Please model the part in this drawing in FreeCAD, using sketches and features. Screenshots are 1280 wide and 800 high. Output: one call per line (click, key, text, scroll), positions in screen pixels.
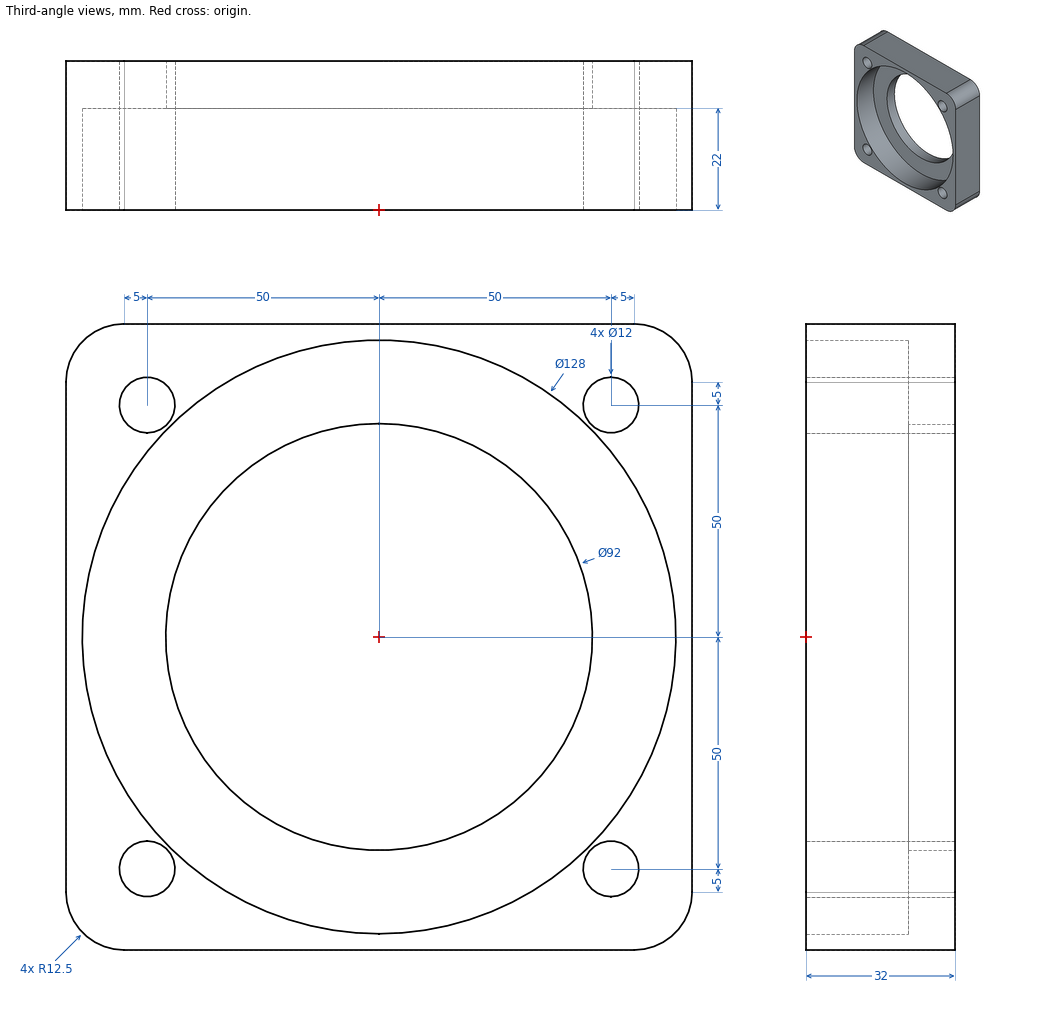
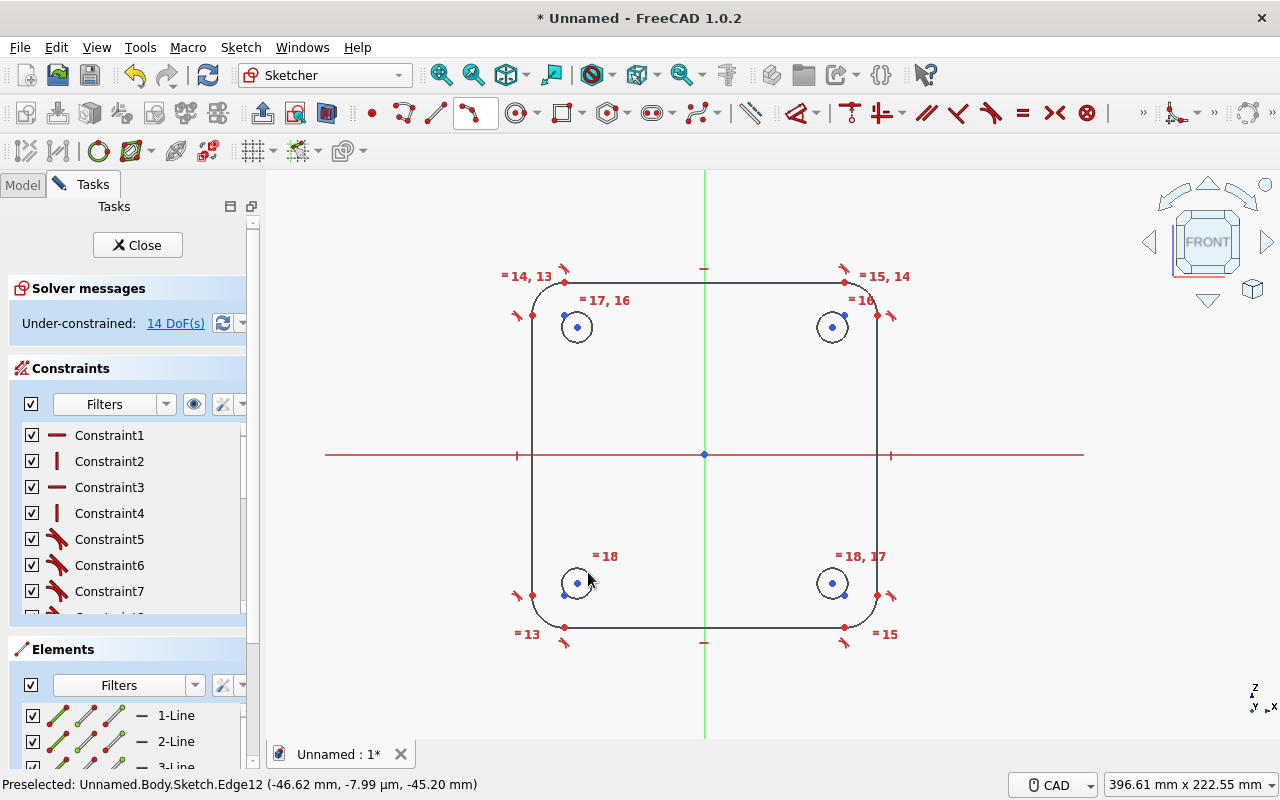
click(833, 327)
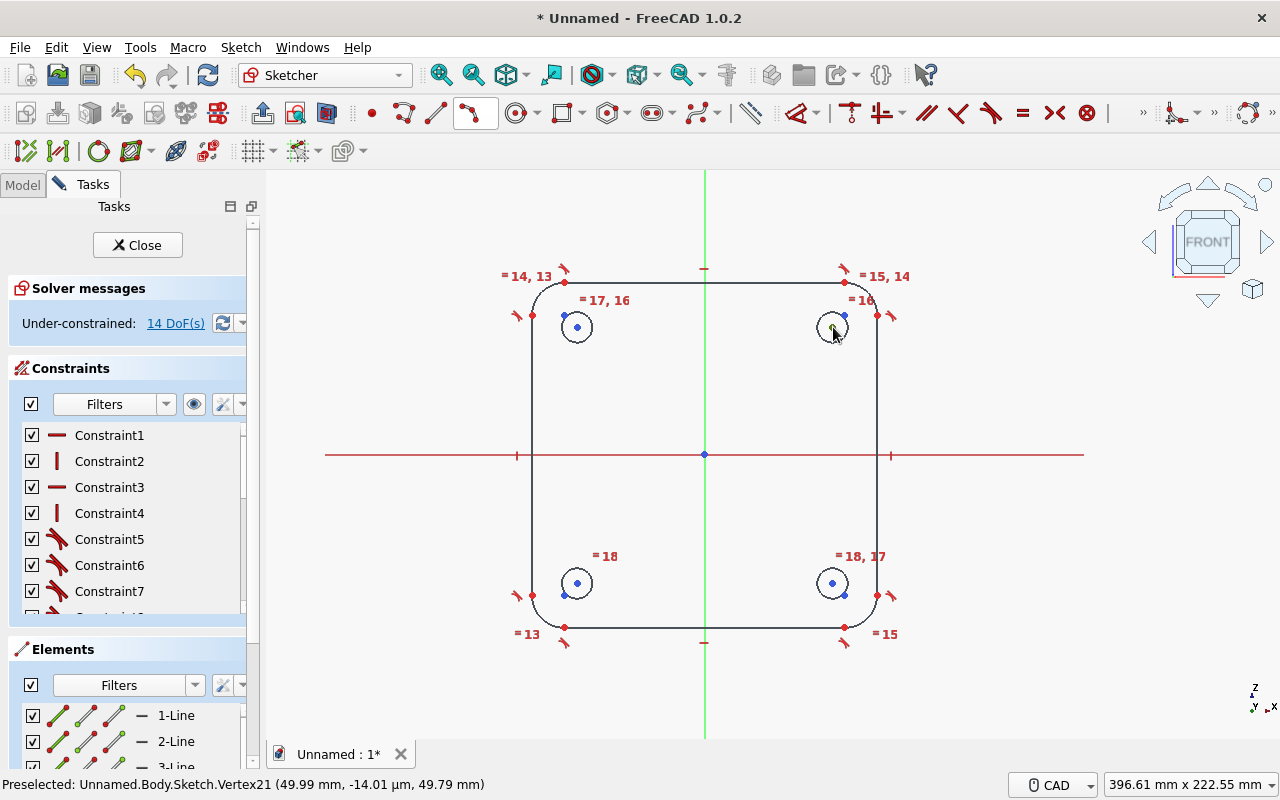
click(577, 327)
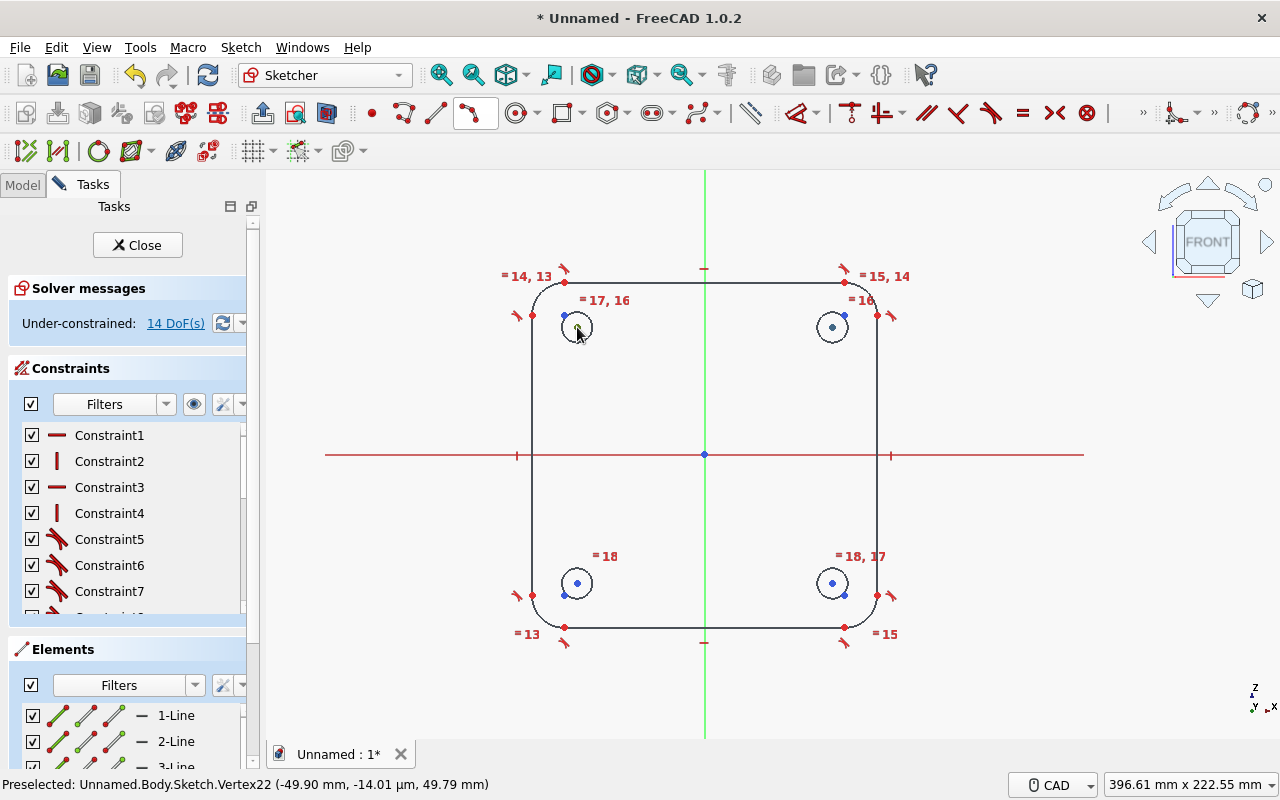
key(h)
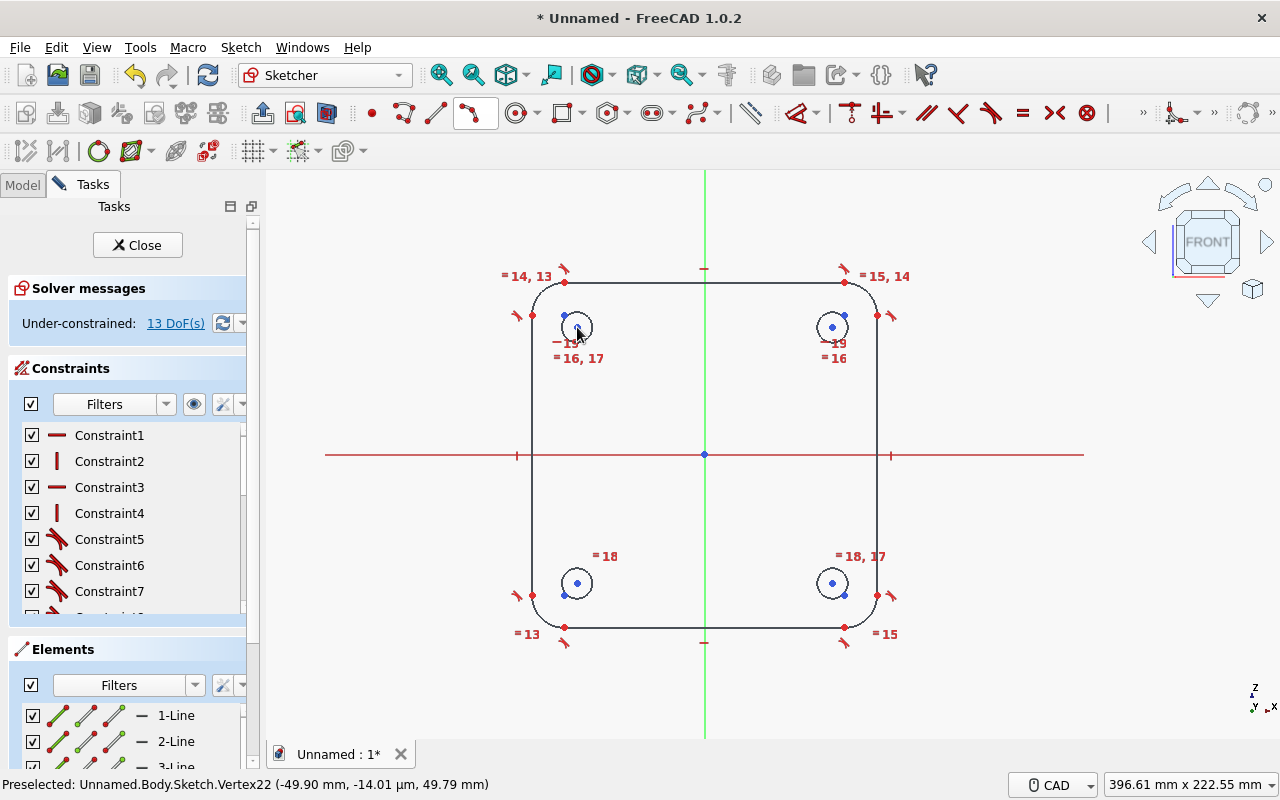
click(833, 327)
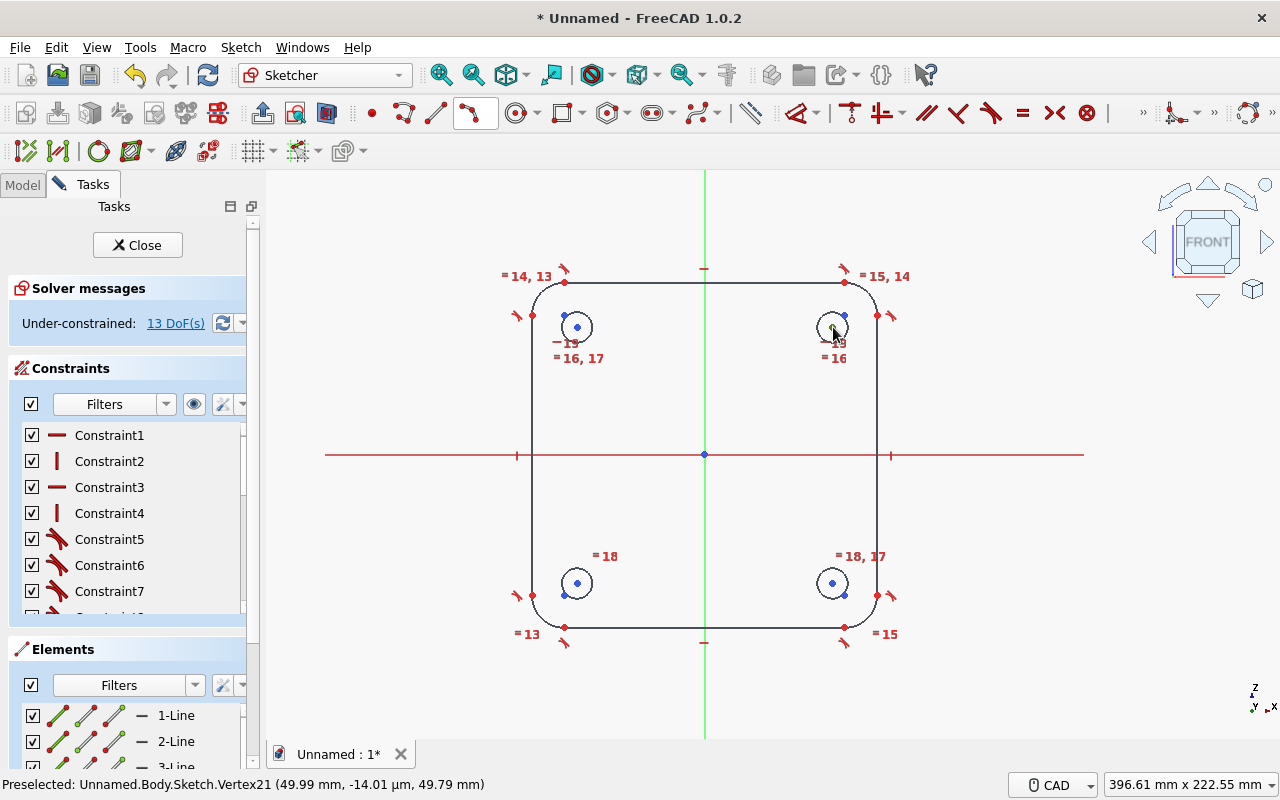
click(833, 583)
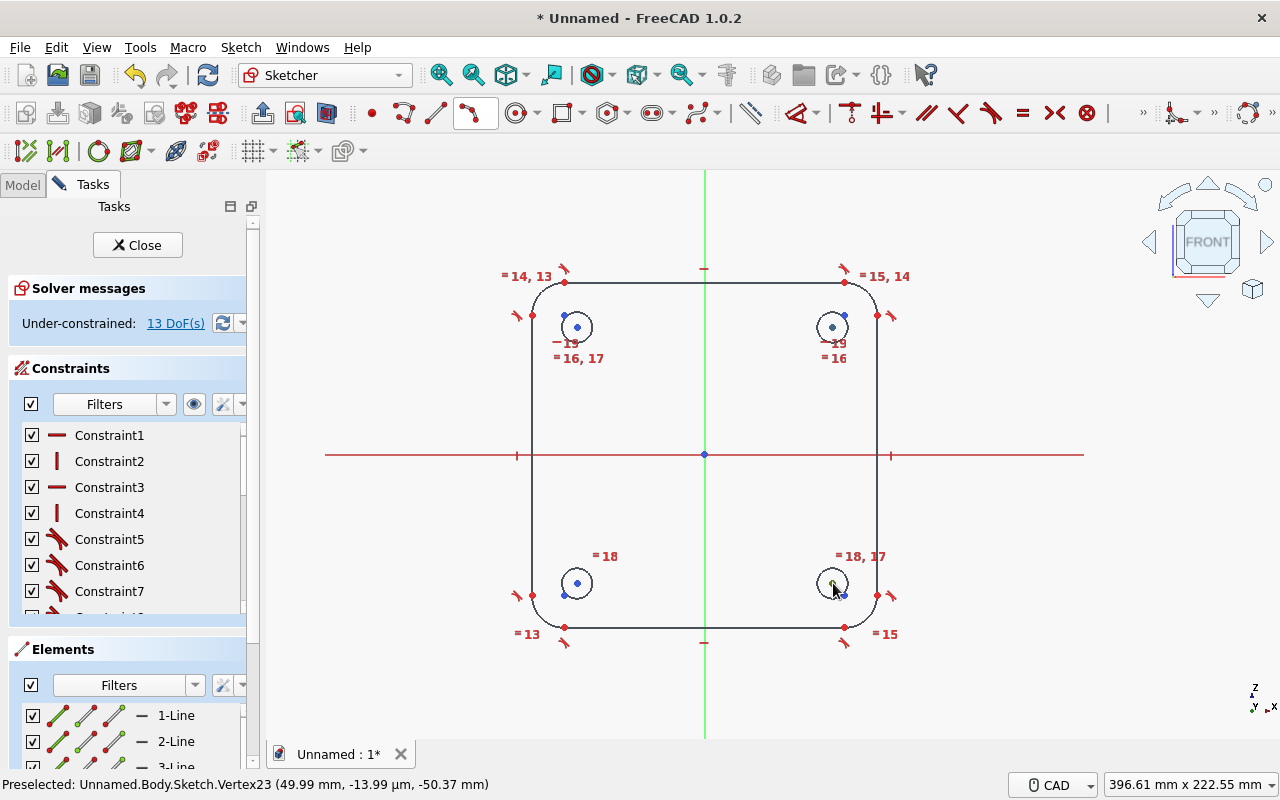
click(904, 114)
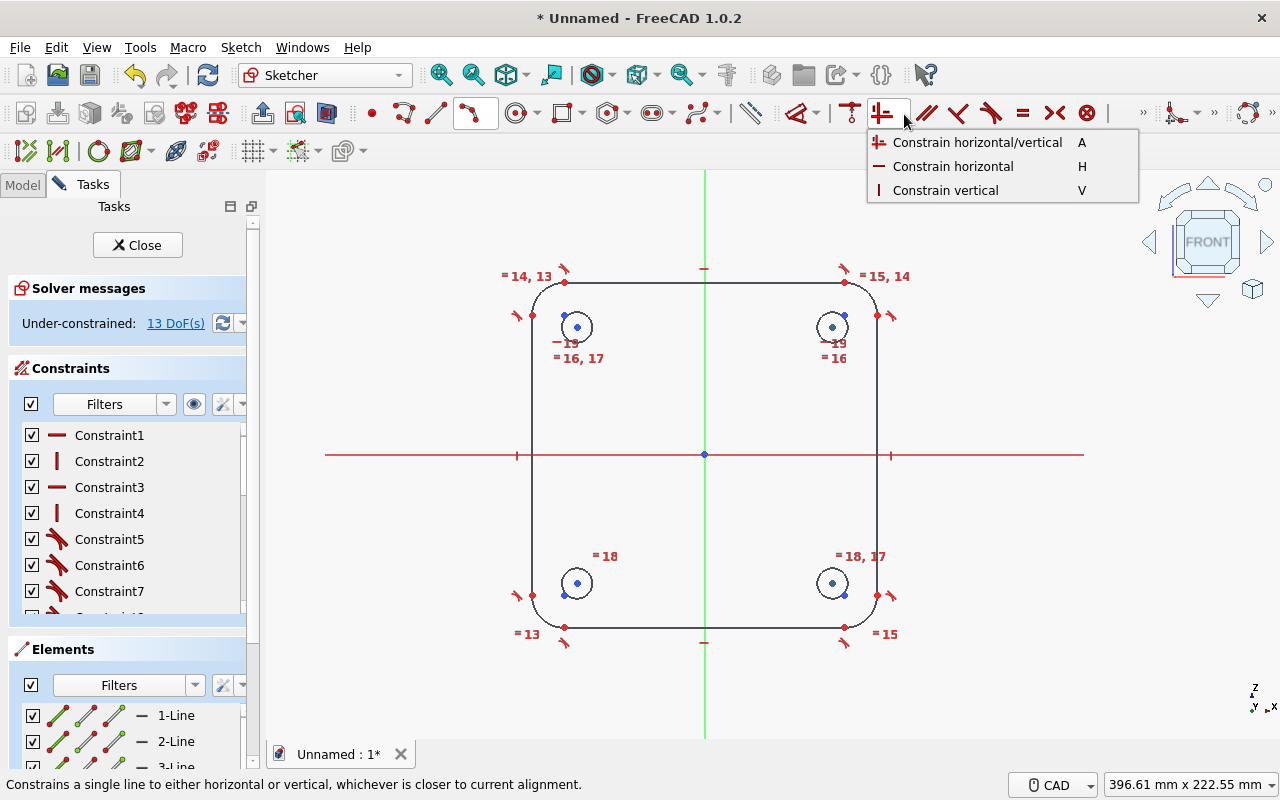
click(1003, 190)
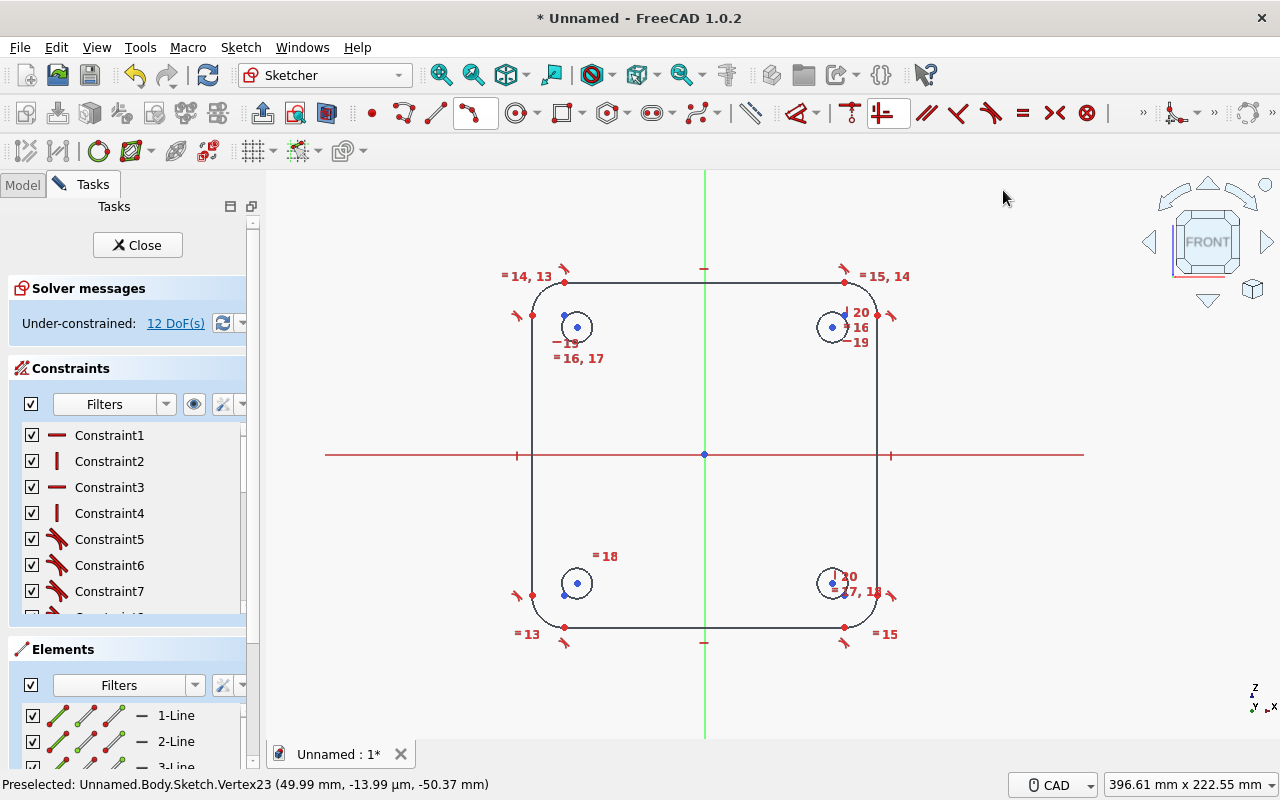
click(577, 327)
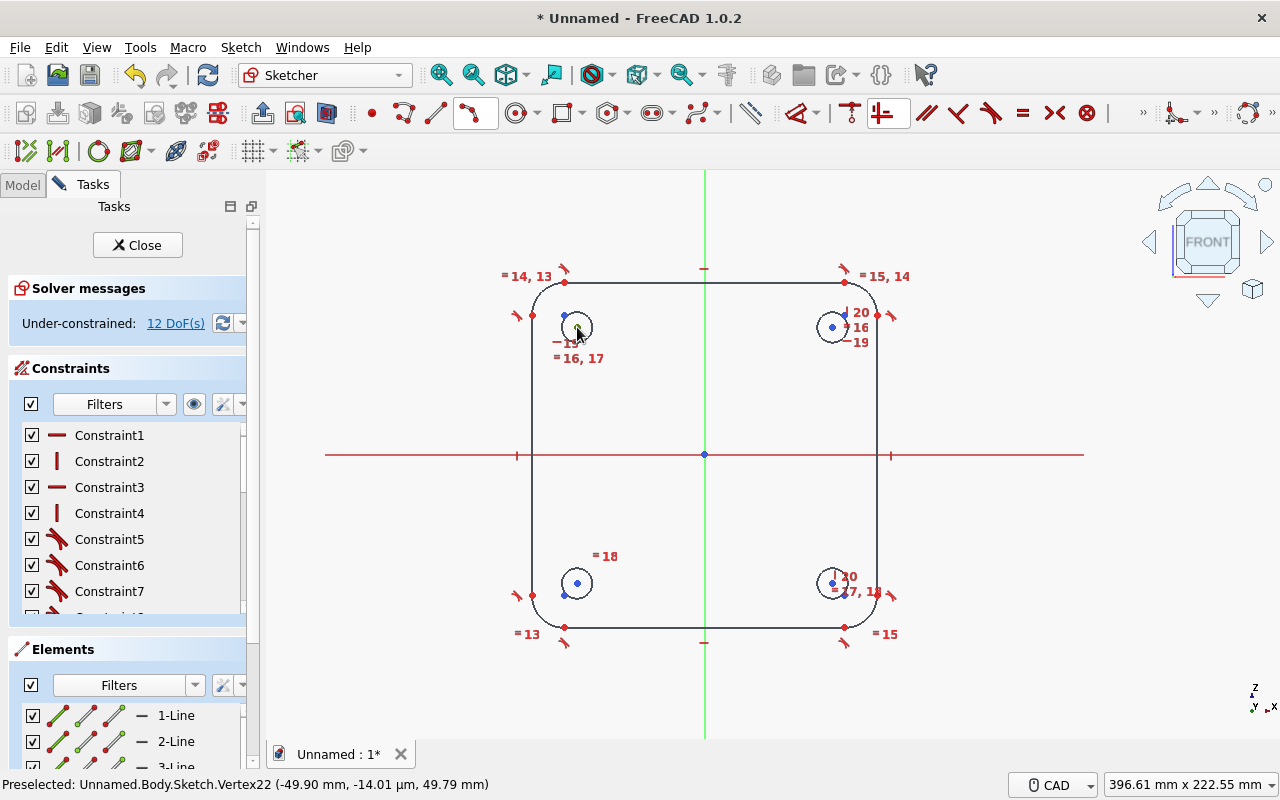
click(577, 583)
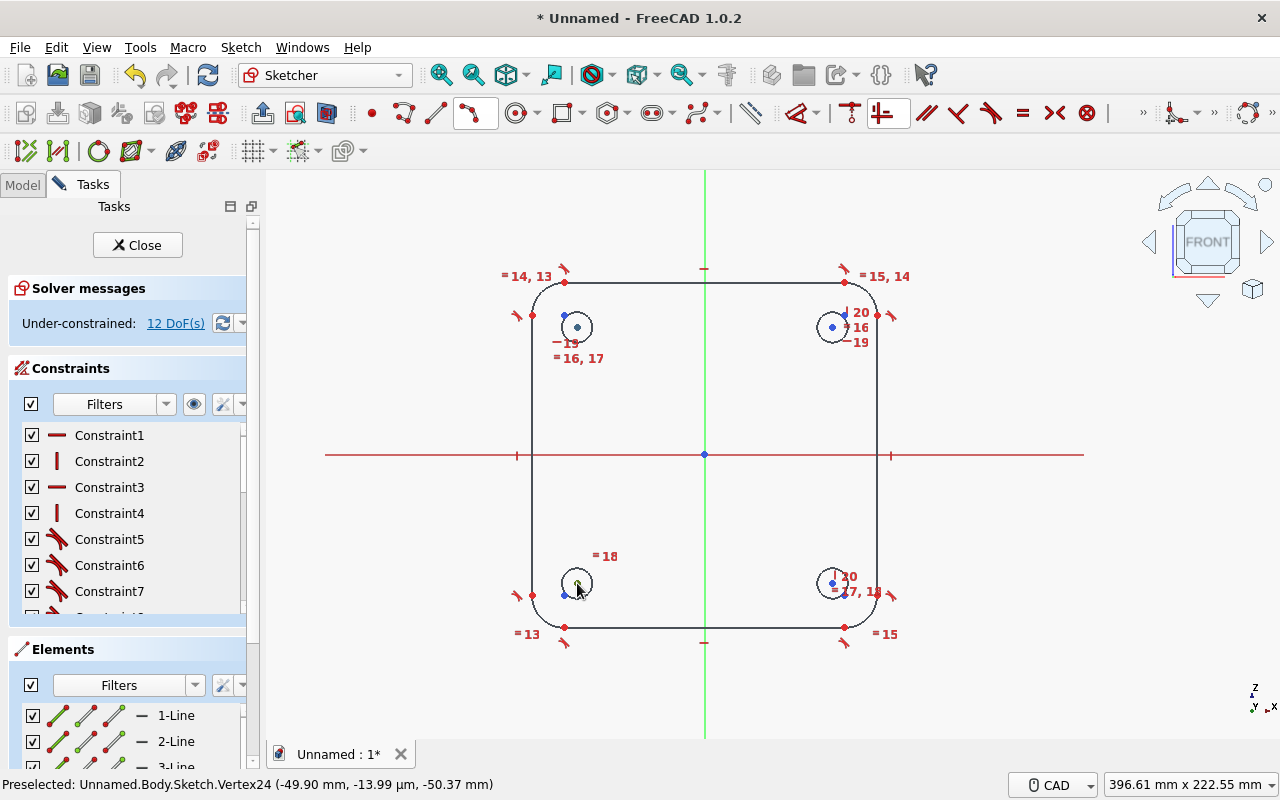
key(v)